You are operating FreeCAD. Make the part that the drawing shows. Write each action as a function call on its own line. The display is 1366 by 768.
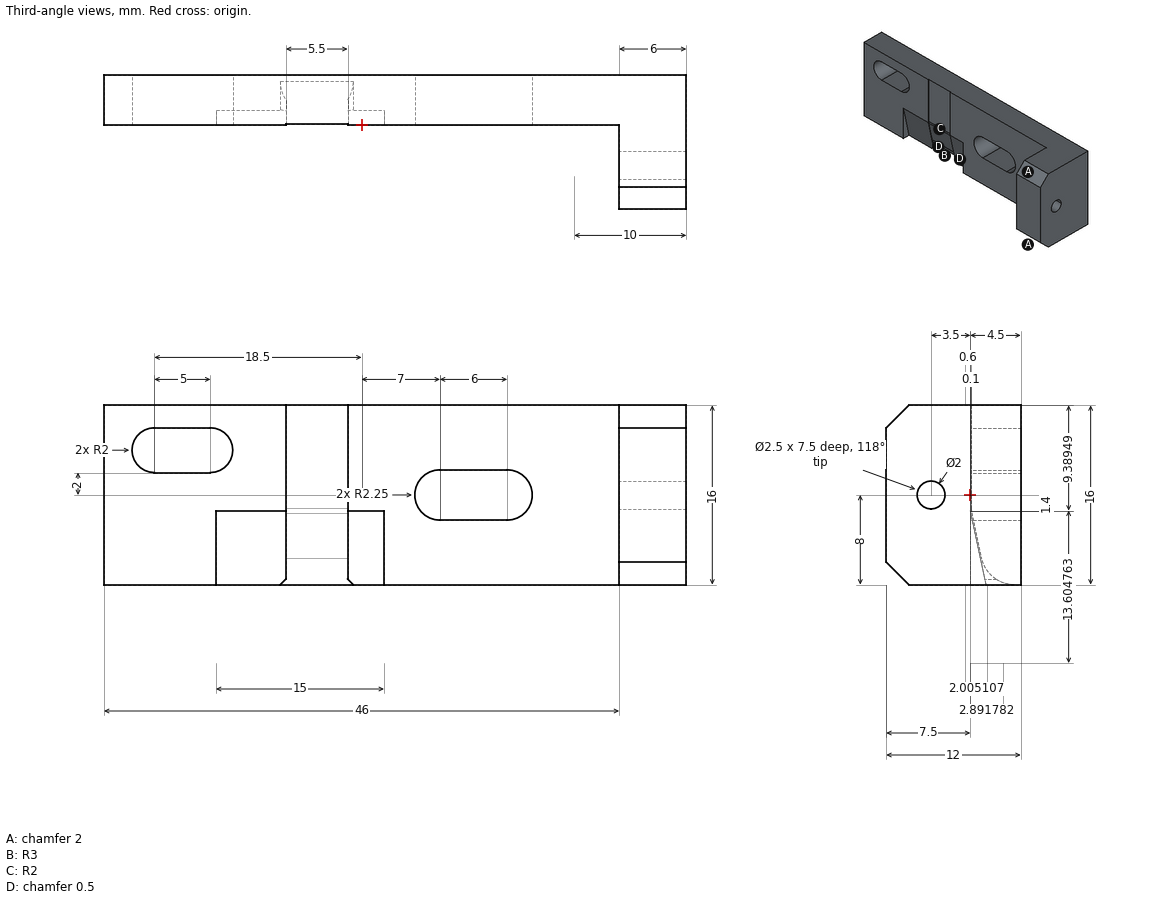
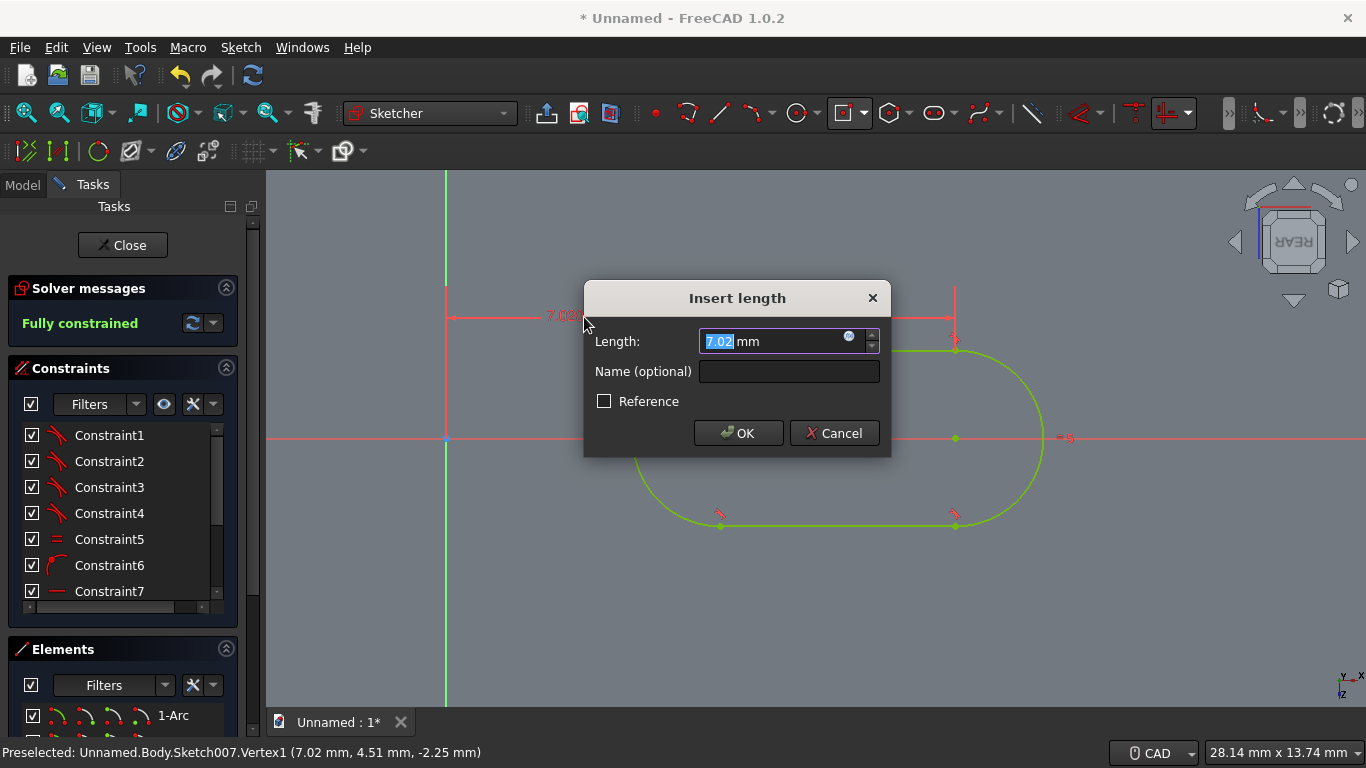
text(7)
key(Return)
key(Escape)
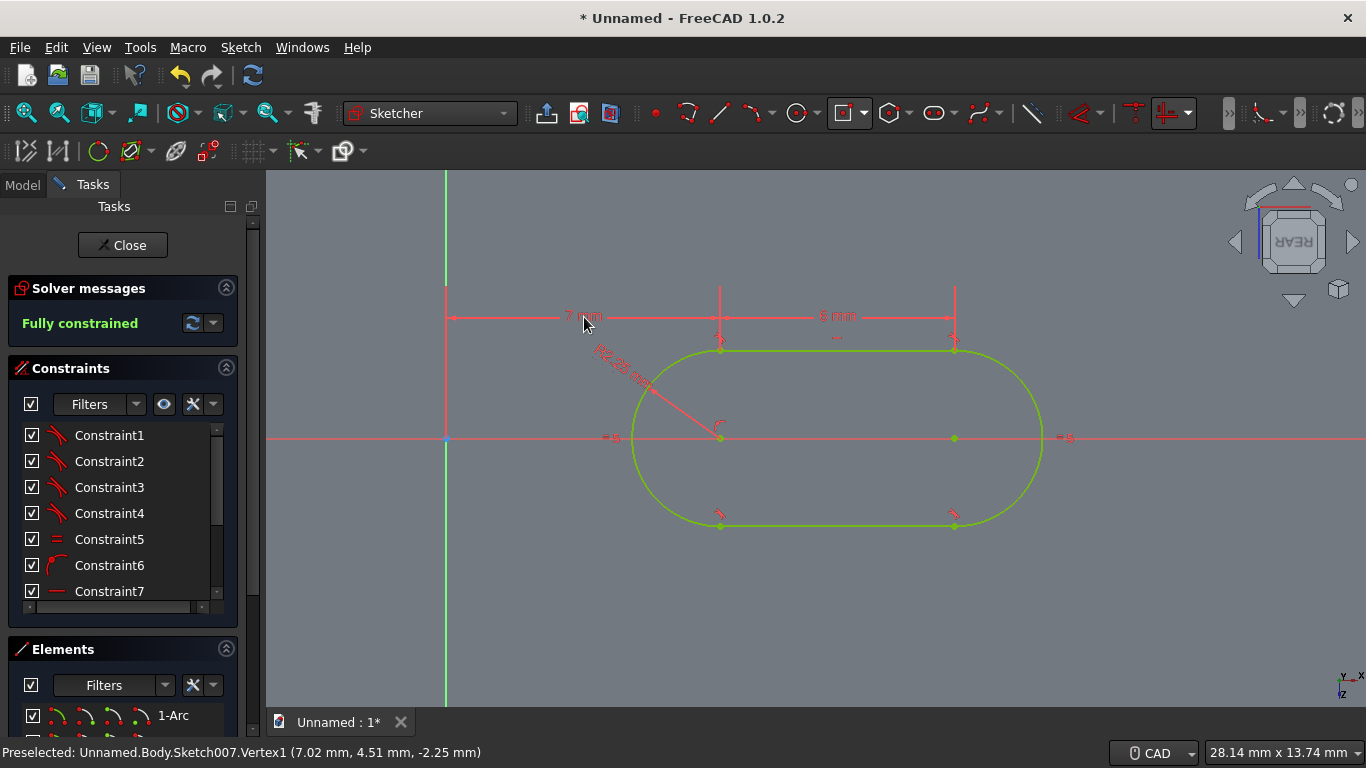
click(123, 245)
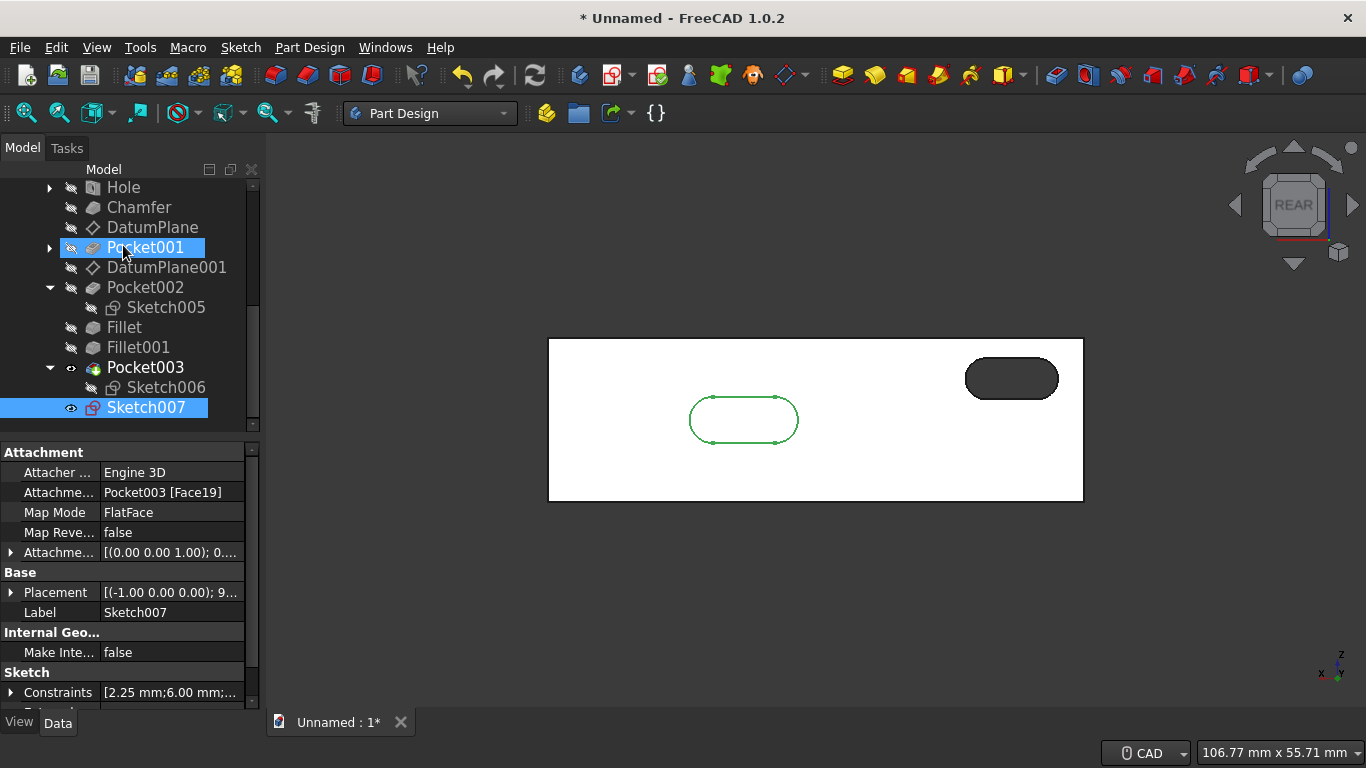
click(1058, 76)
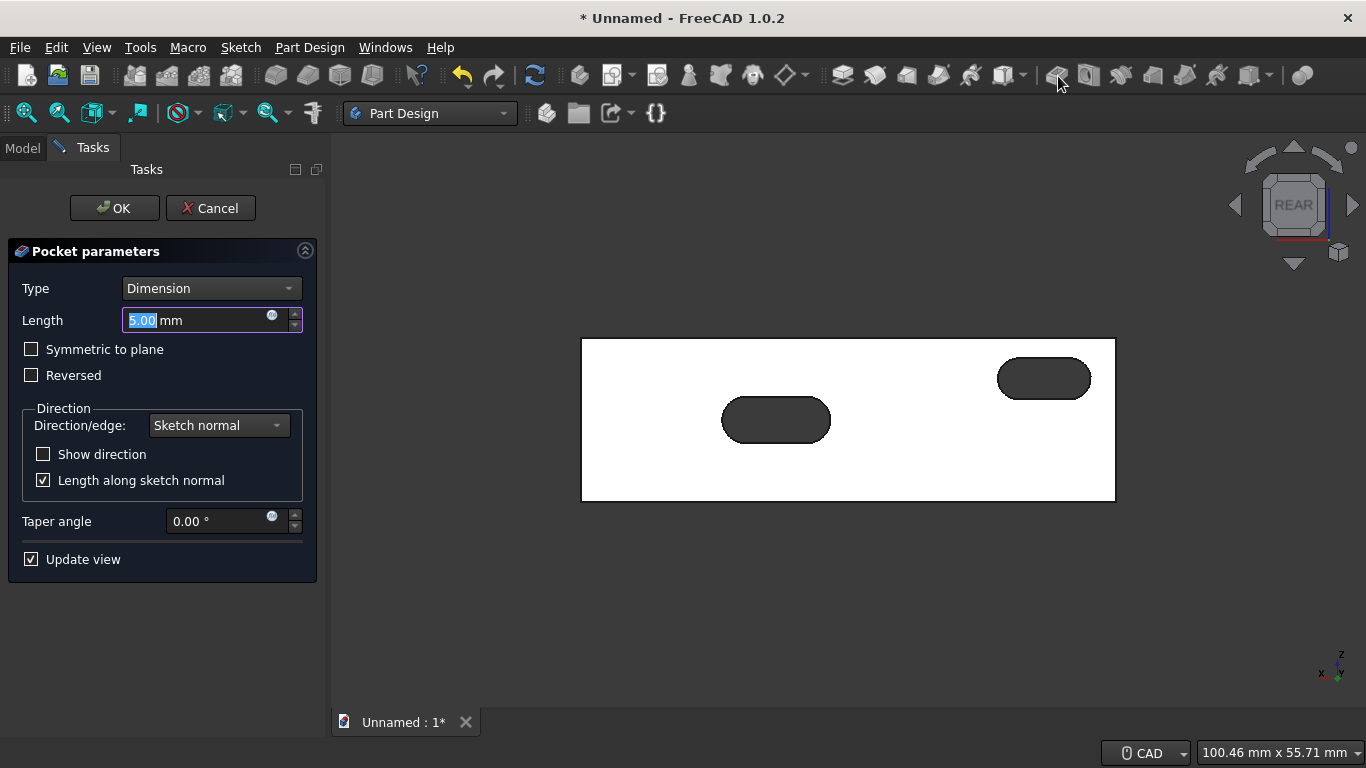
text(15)
key(Tab)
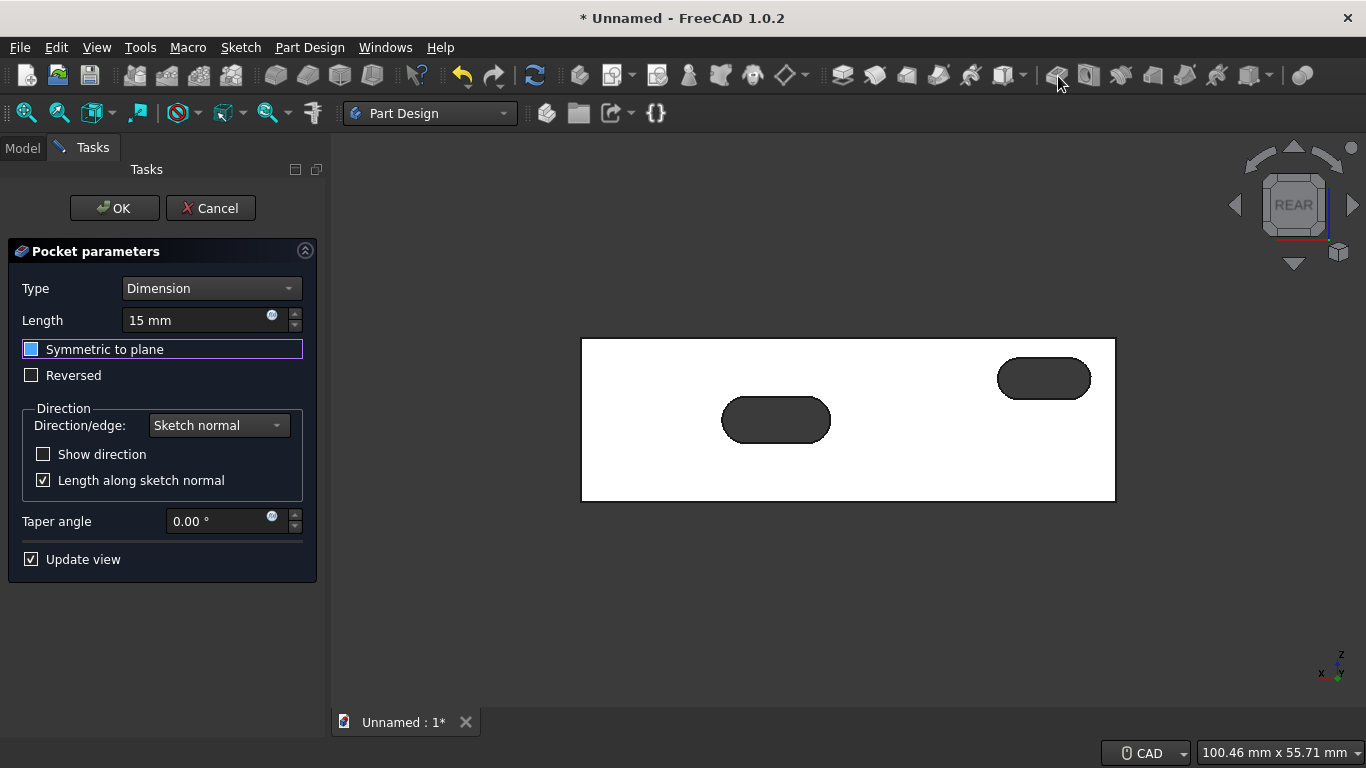
click(115, 208)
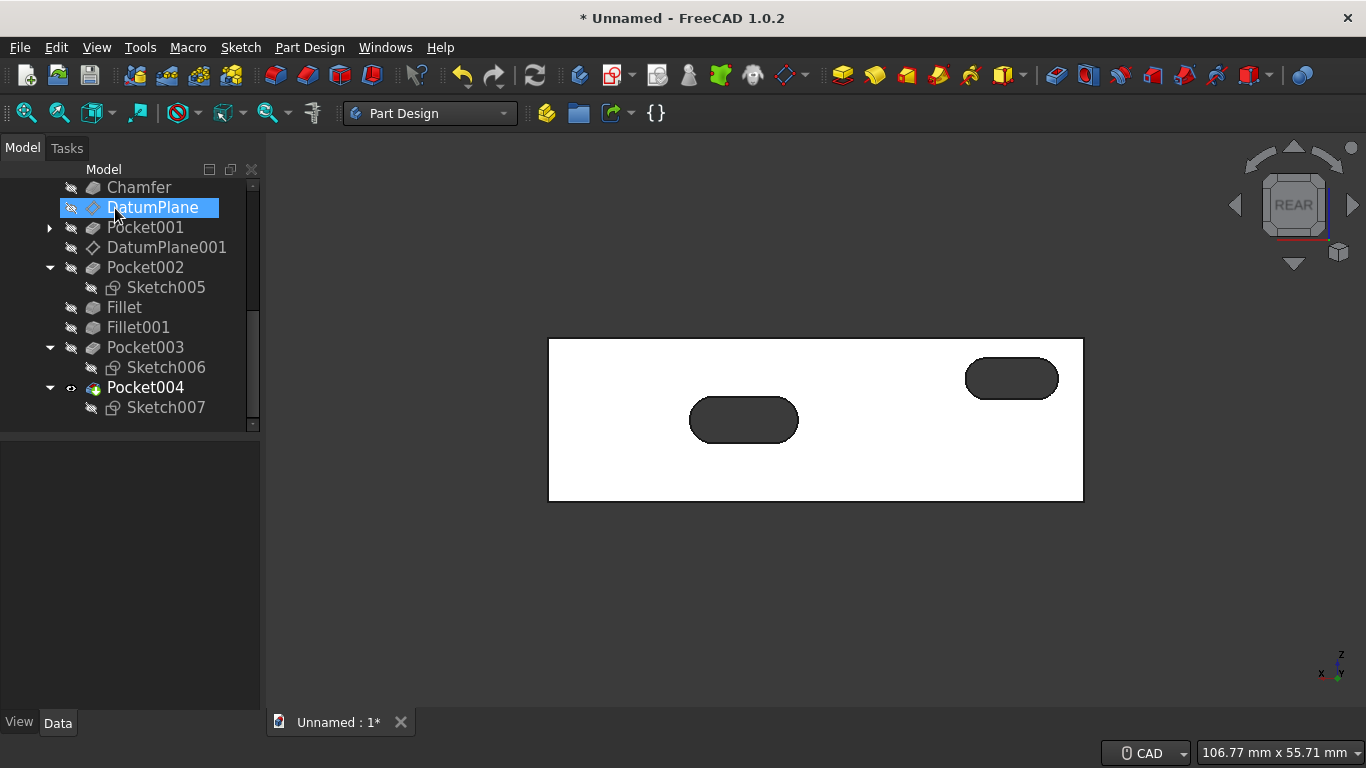
key(0)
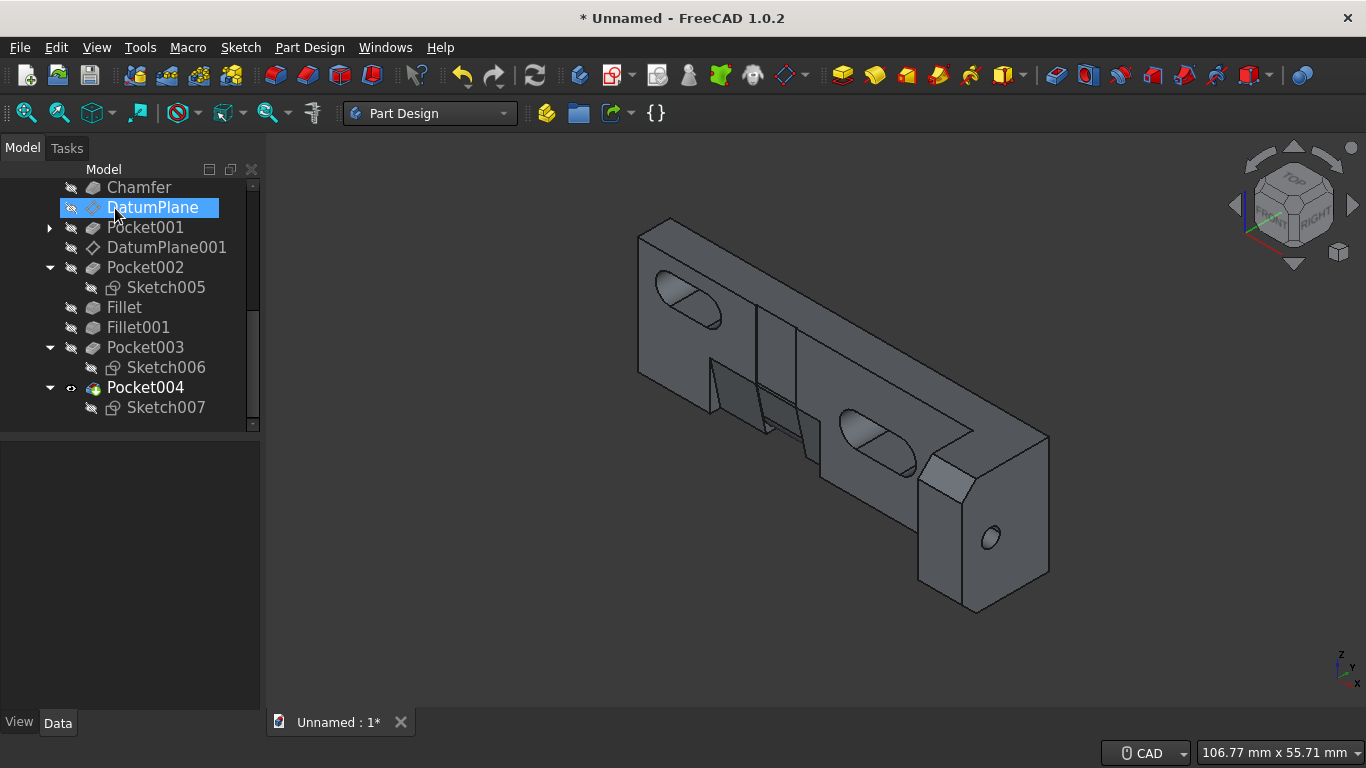
key(2)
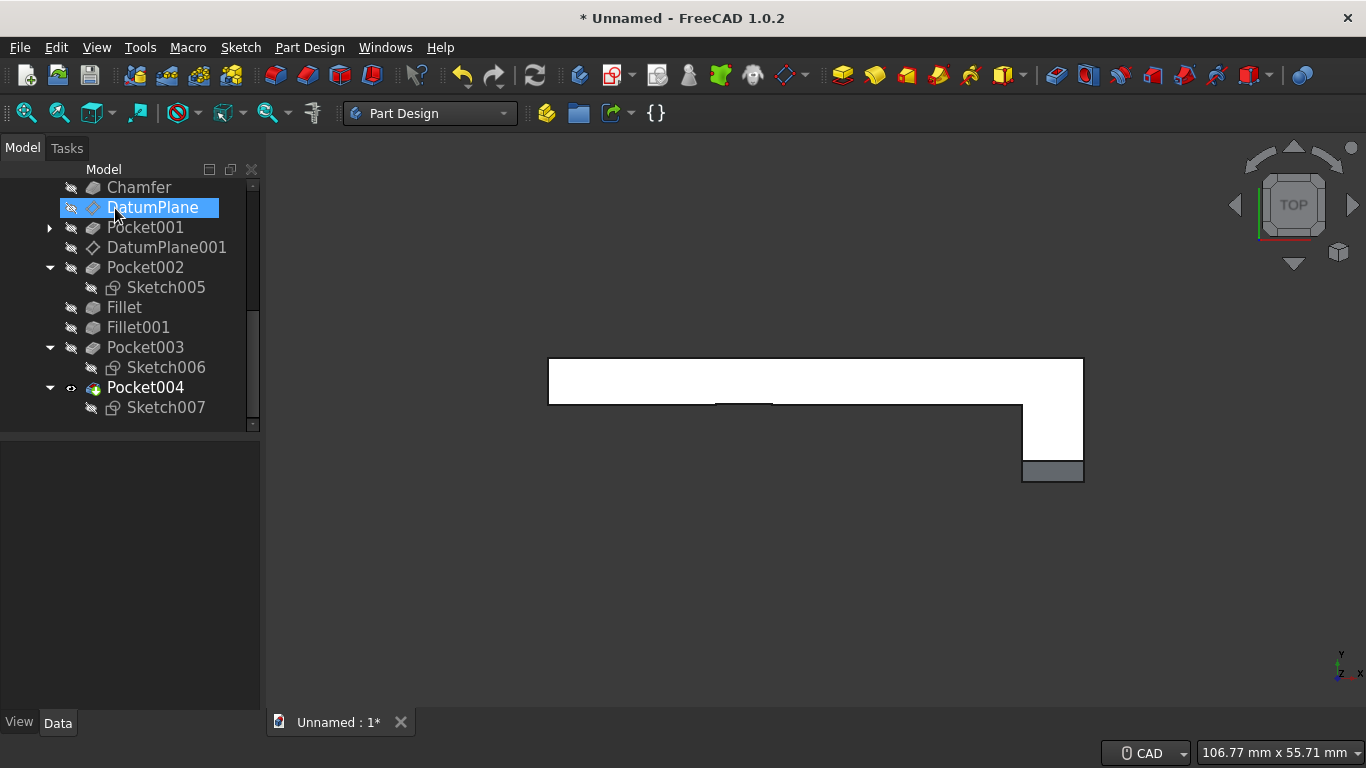
key(1)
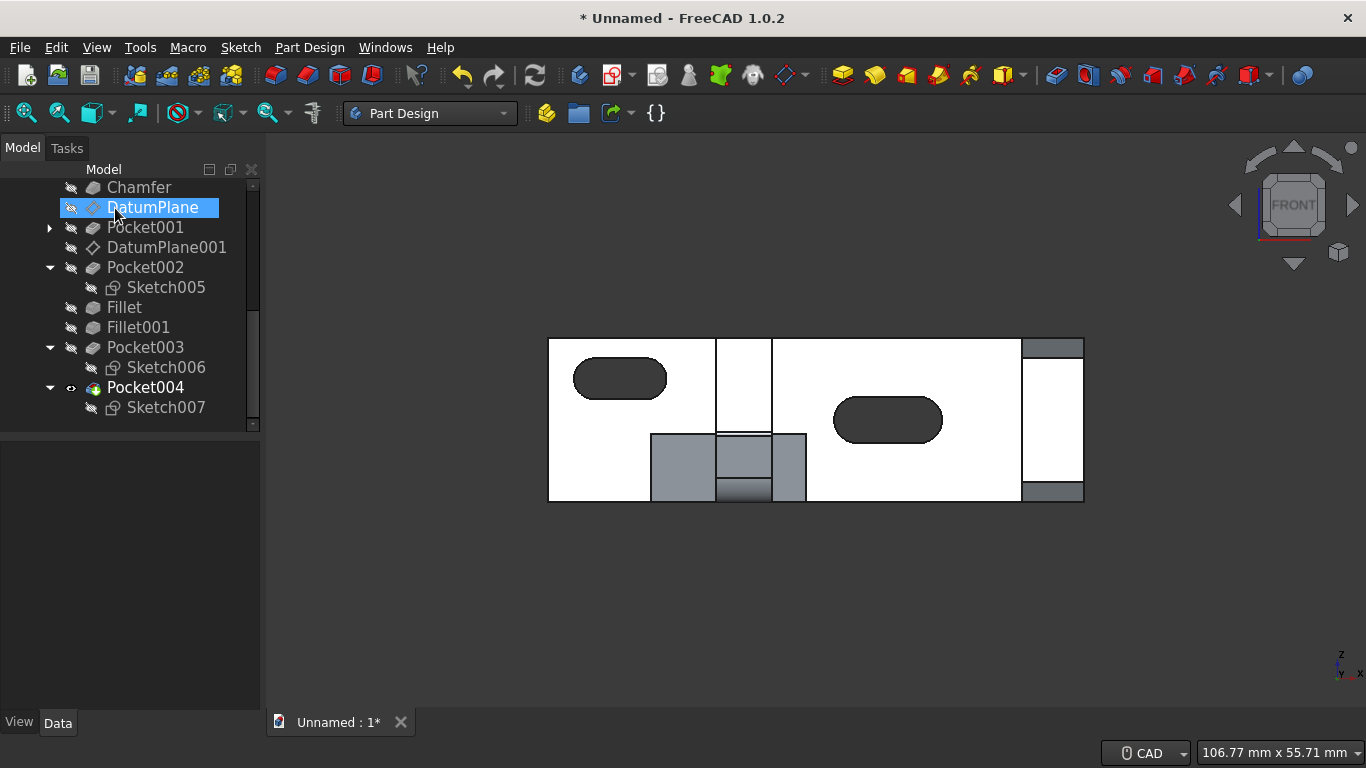
key(3)